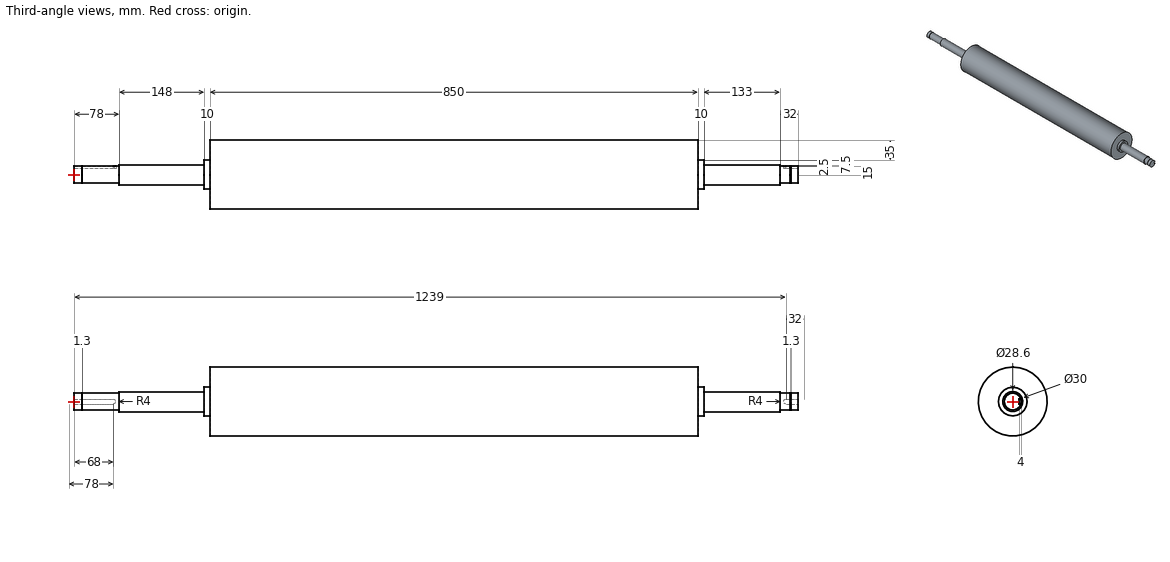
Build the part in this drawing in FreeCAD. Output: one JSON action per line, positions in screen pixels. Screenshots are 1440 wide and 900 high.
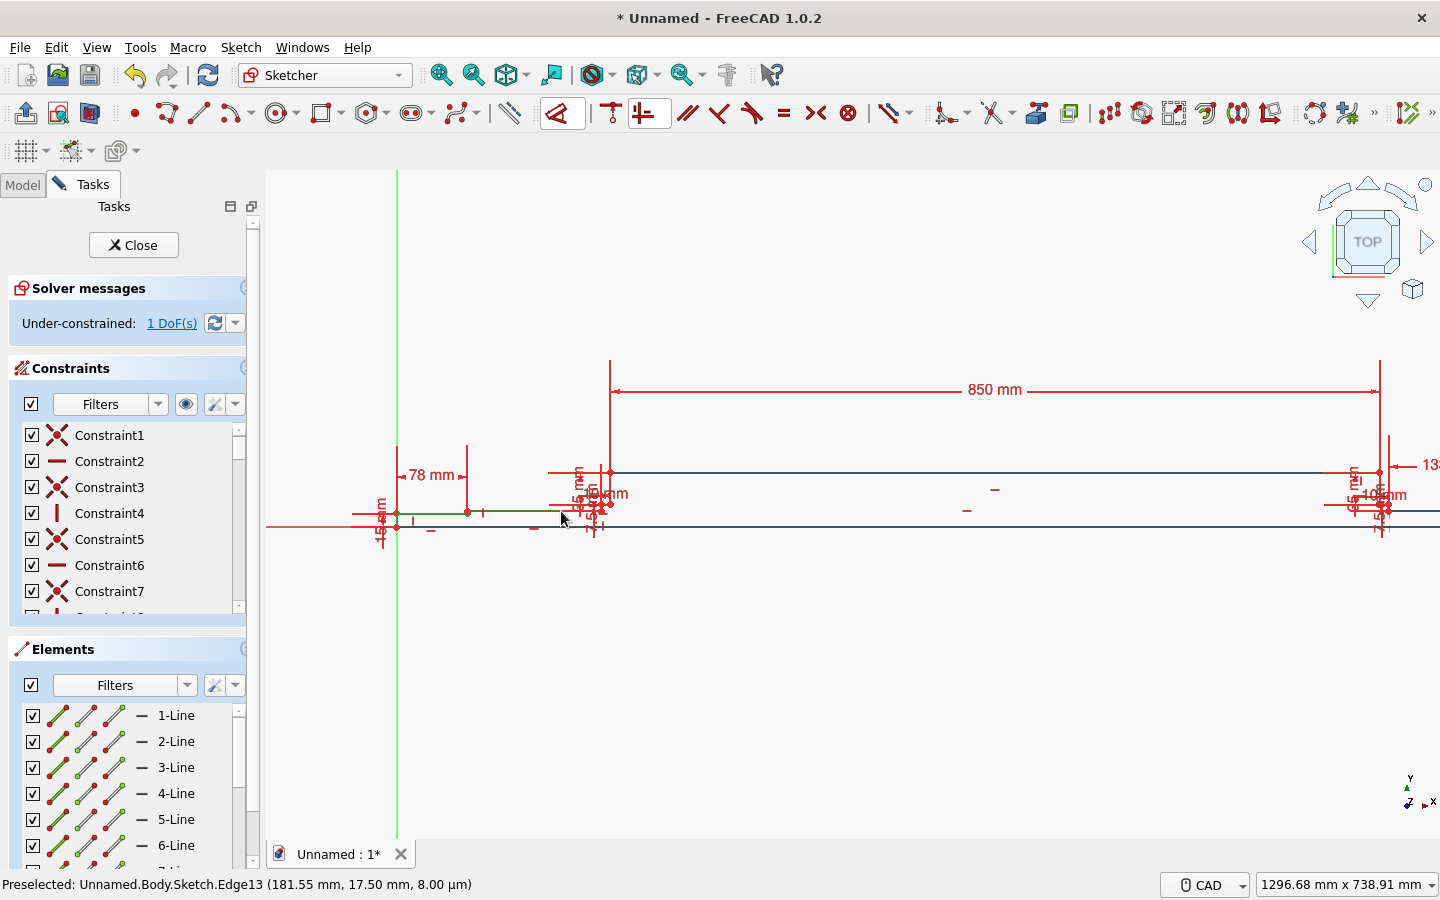
{"action": "key", "text": "l"}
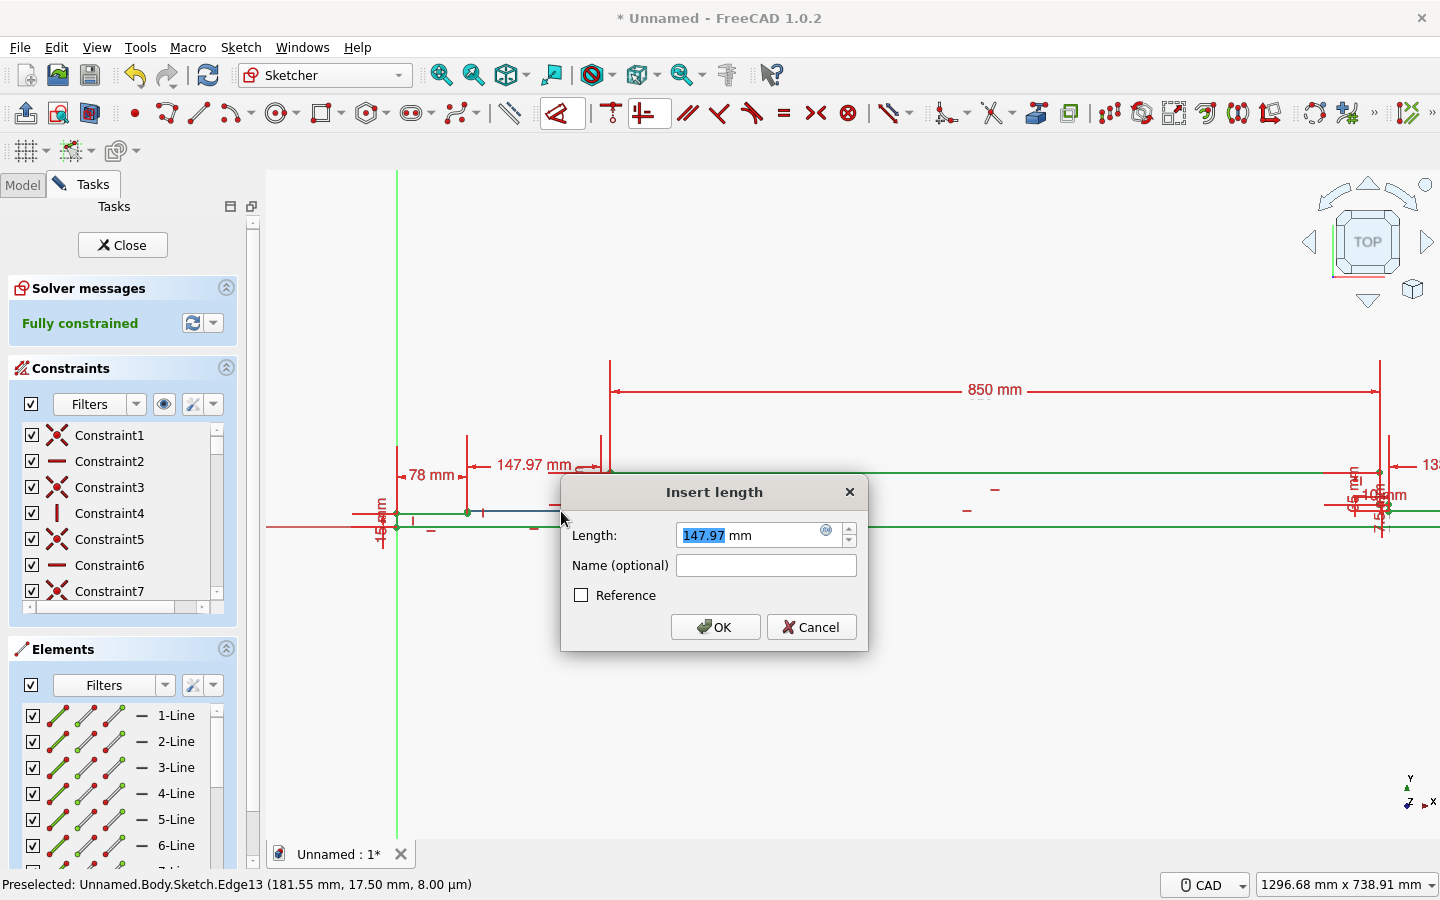
{"action": "type", "text": "148"}
{"action": "key", "text": "Return"}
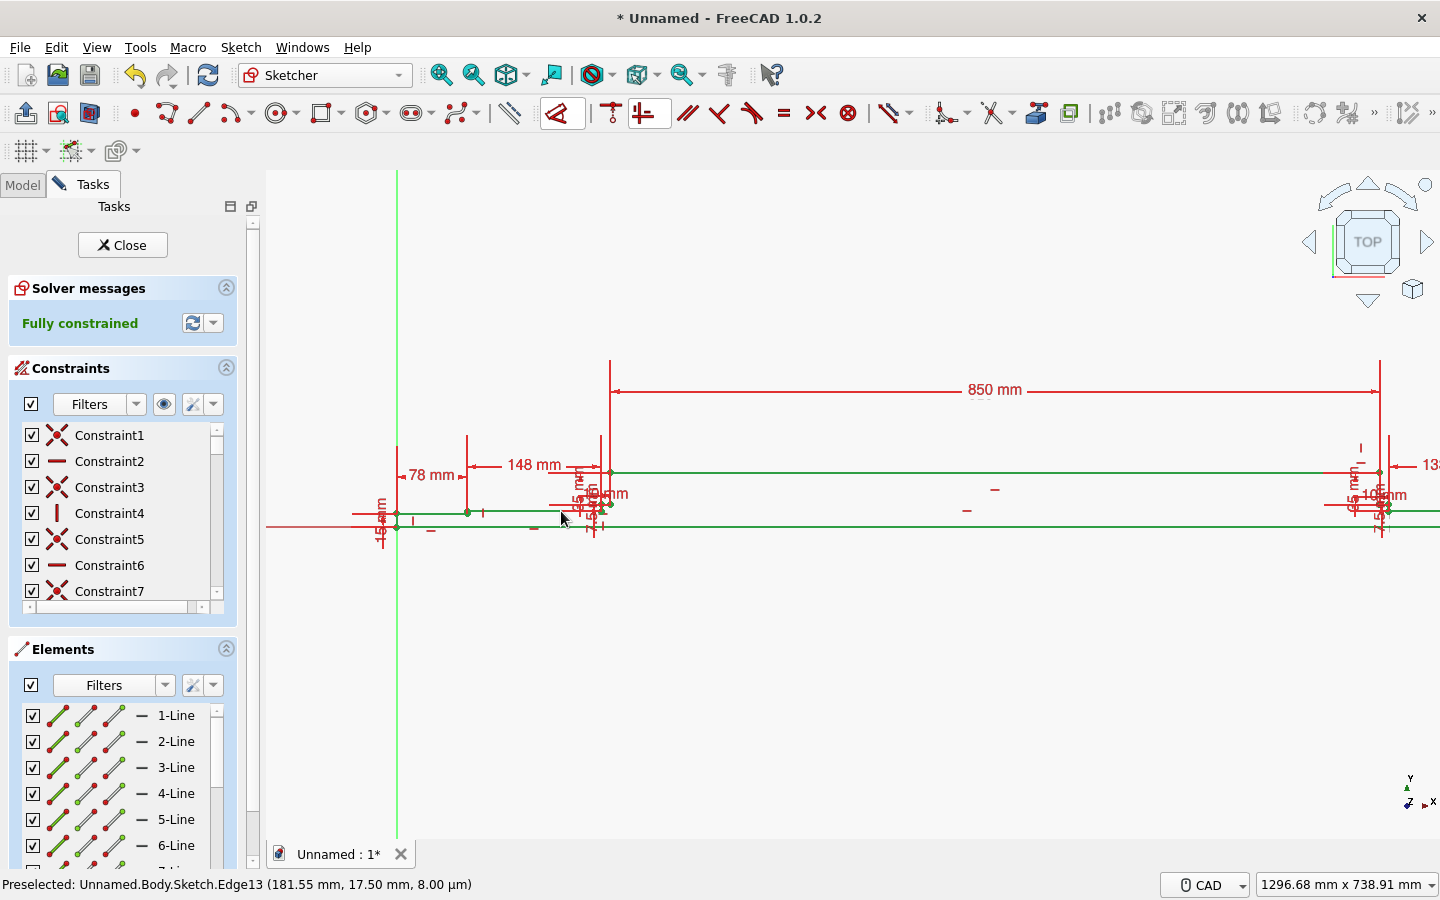
{"action": "left_click", "coordinate": [123, 245]}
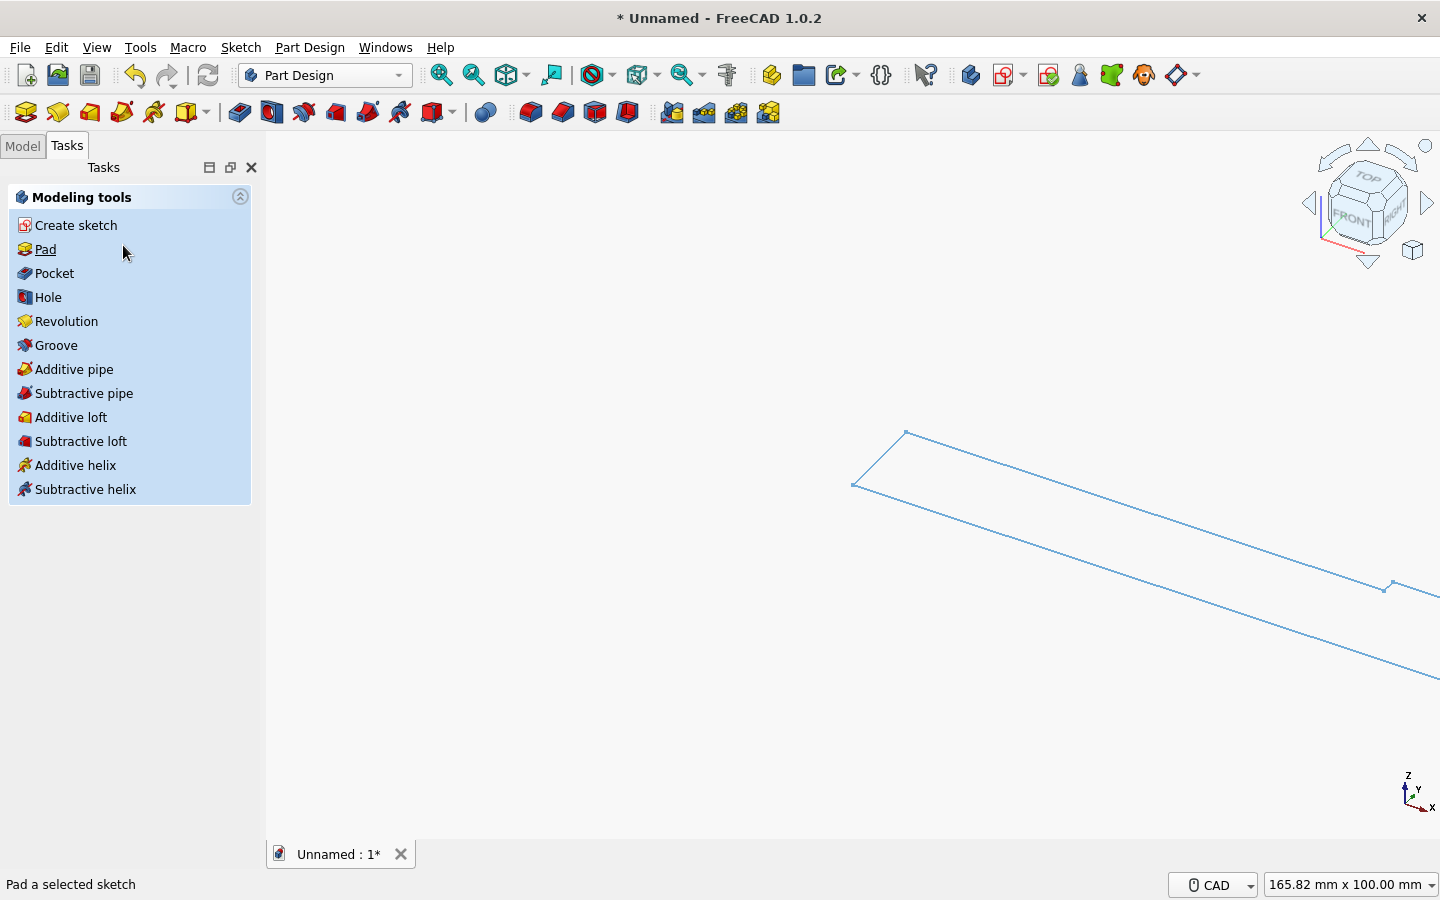
{"action": "left_click", "coordinate": [58, 112]}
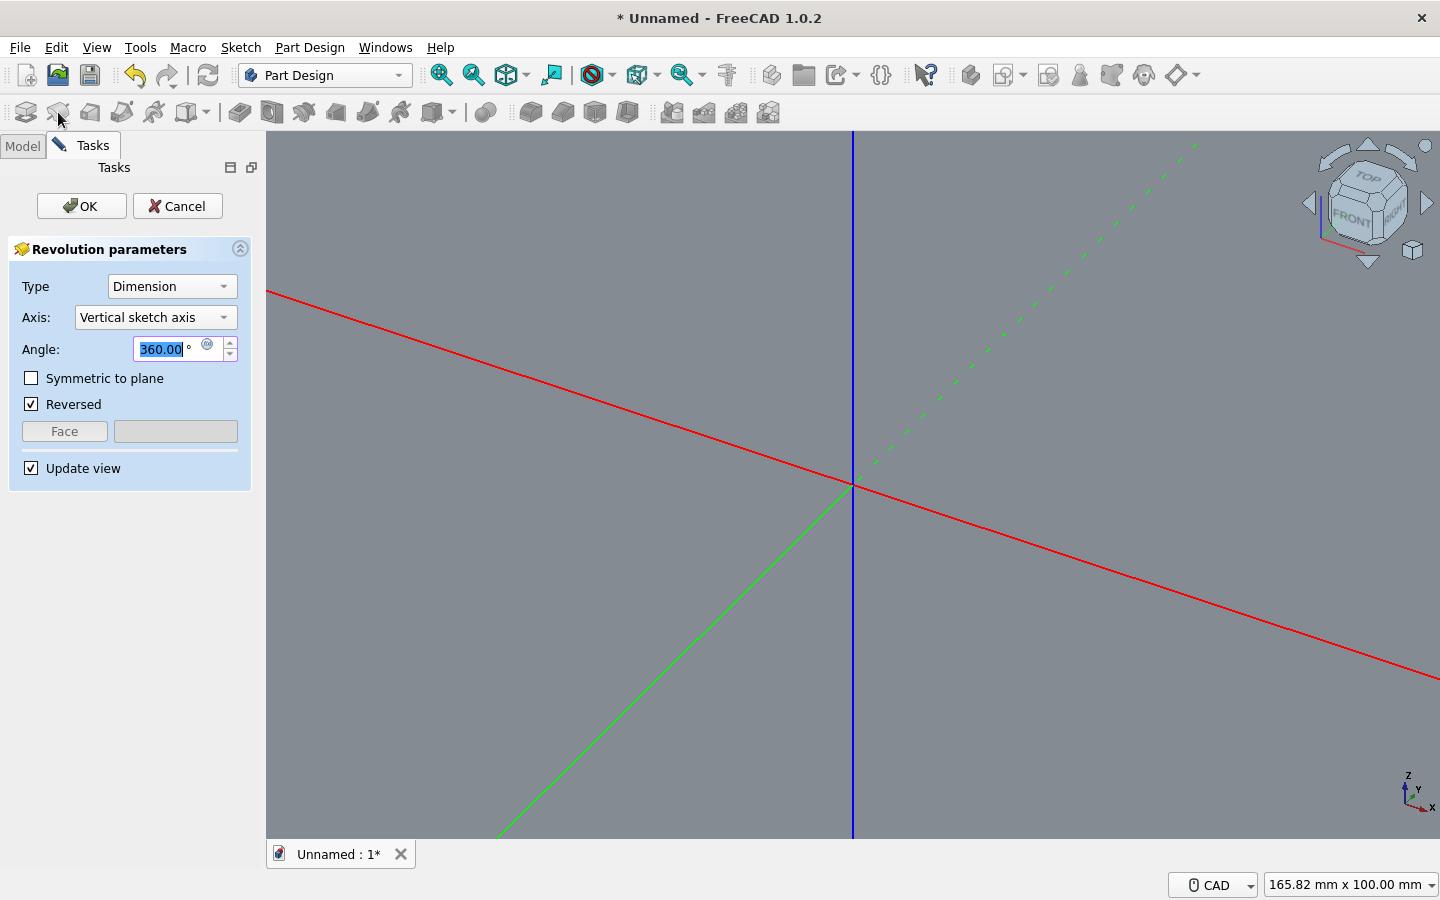
{"action": "left_click", "coordinate": [156, 318]}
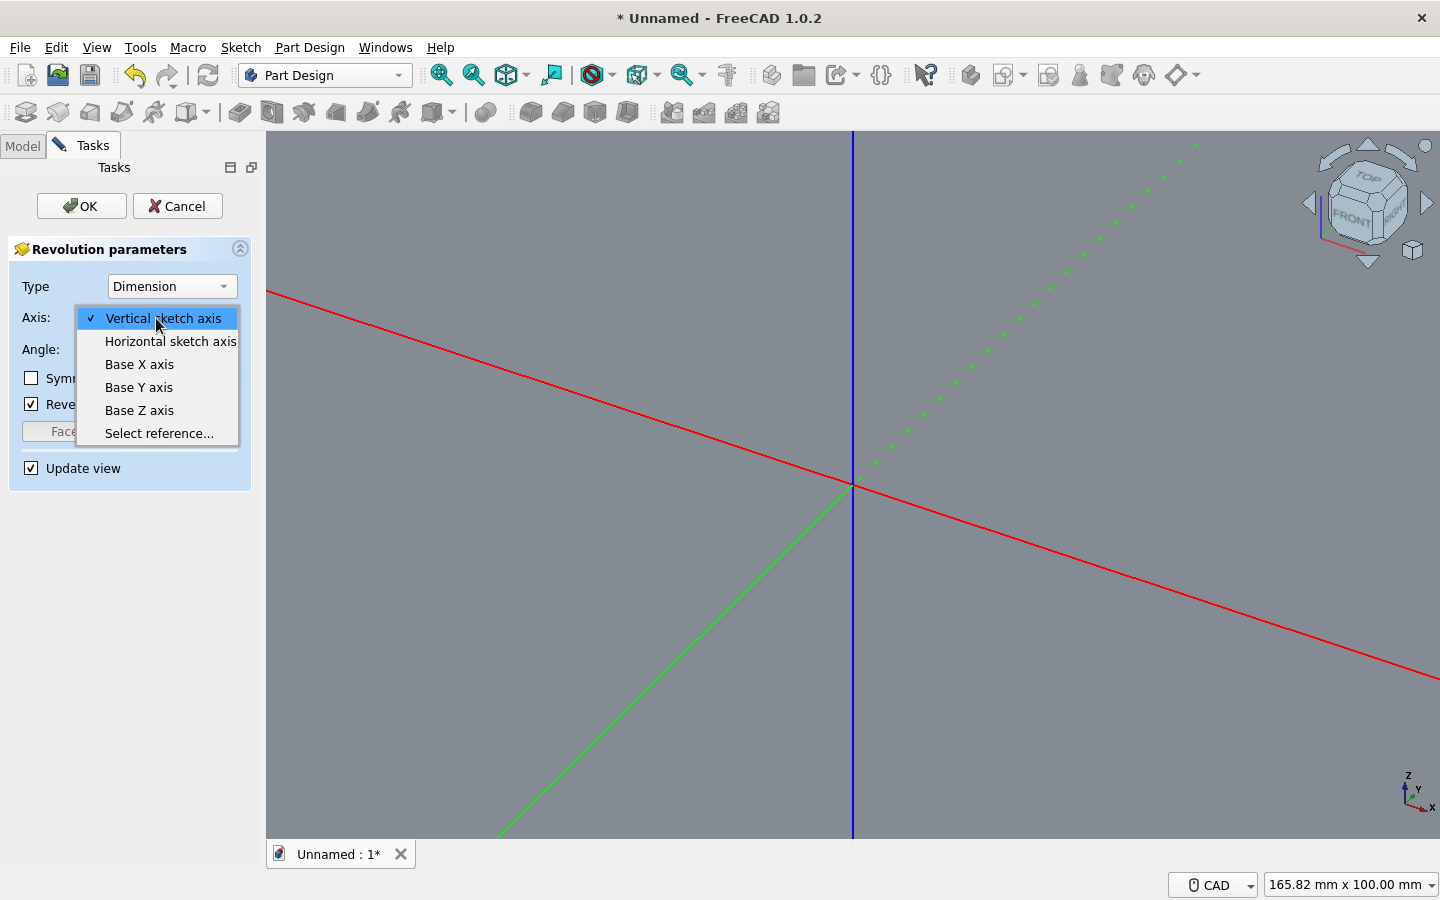
{"action": "left_click", "coordinate": [156, 342]}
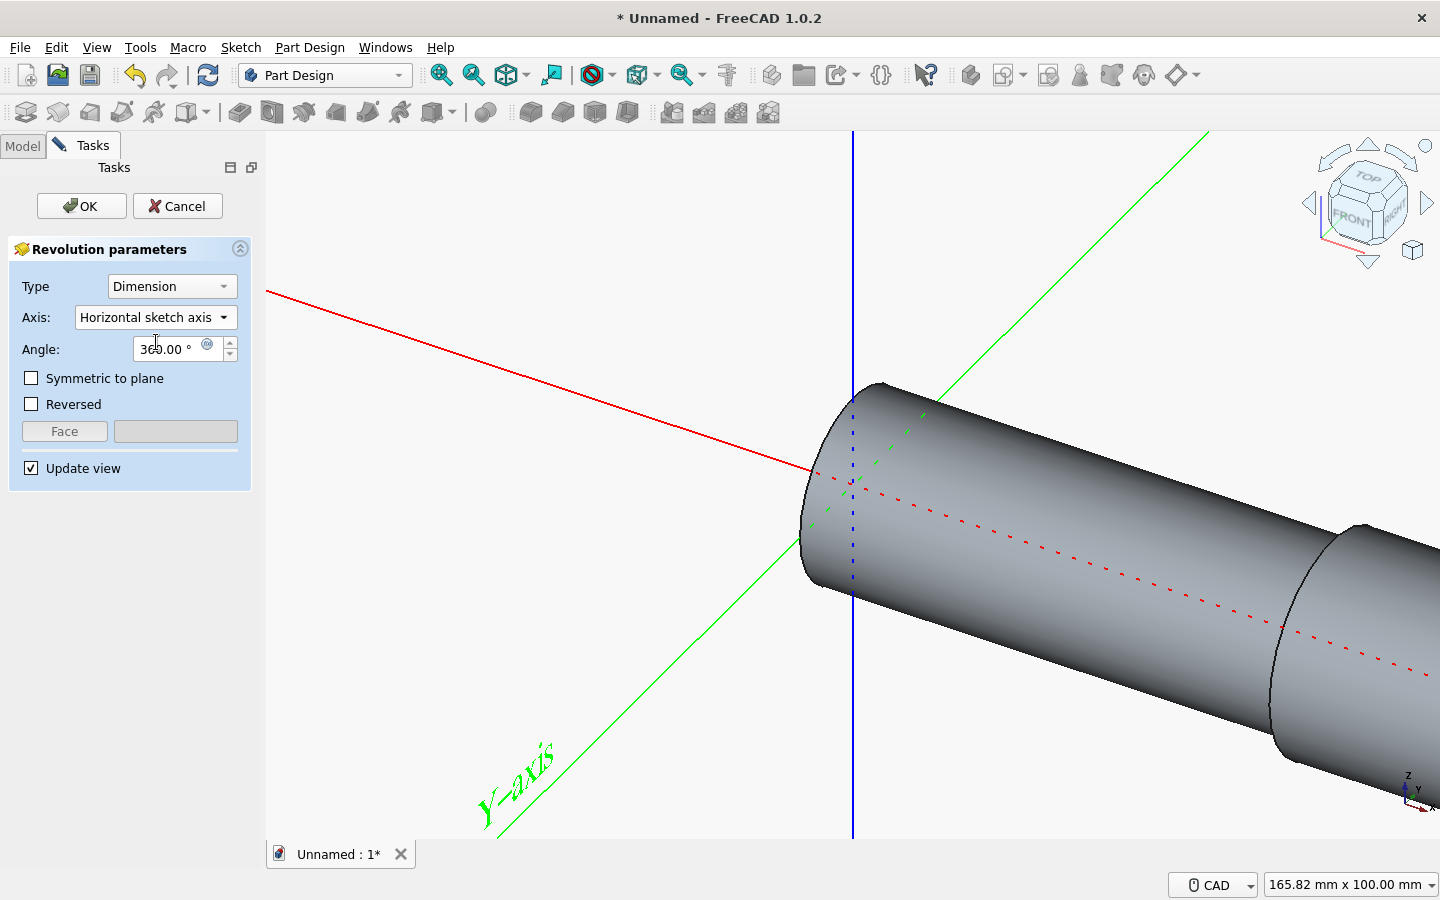
{"action": "left_click", "coordinate": [82, 206]}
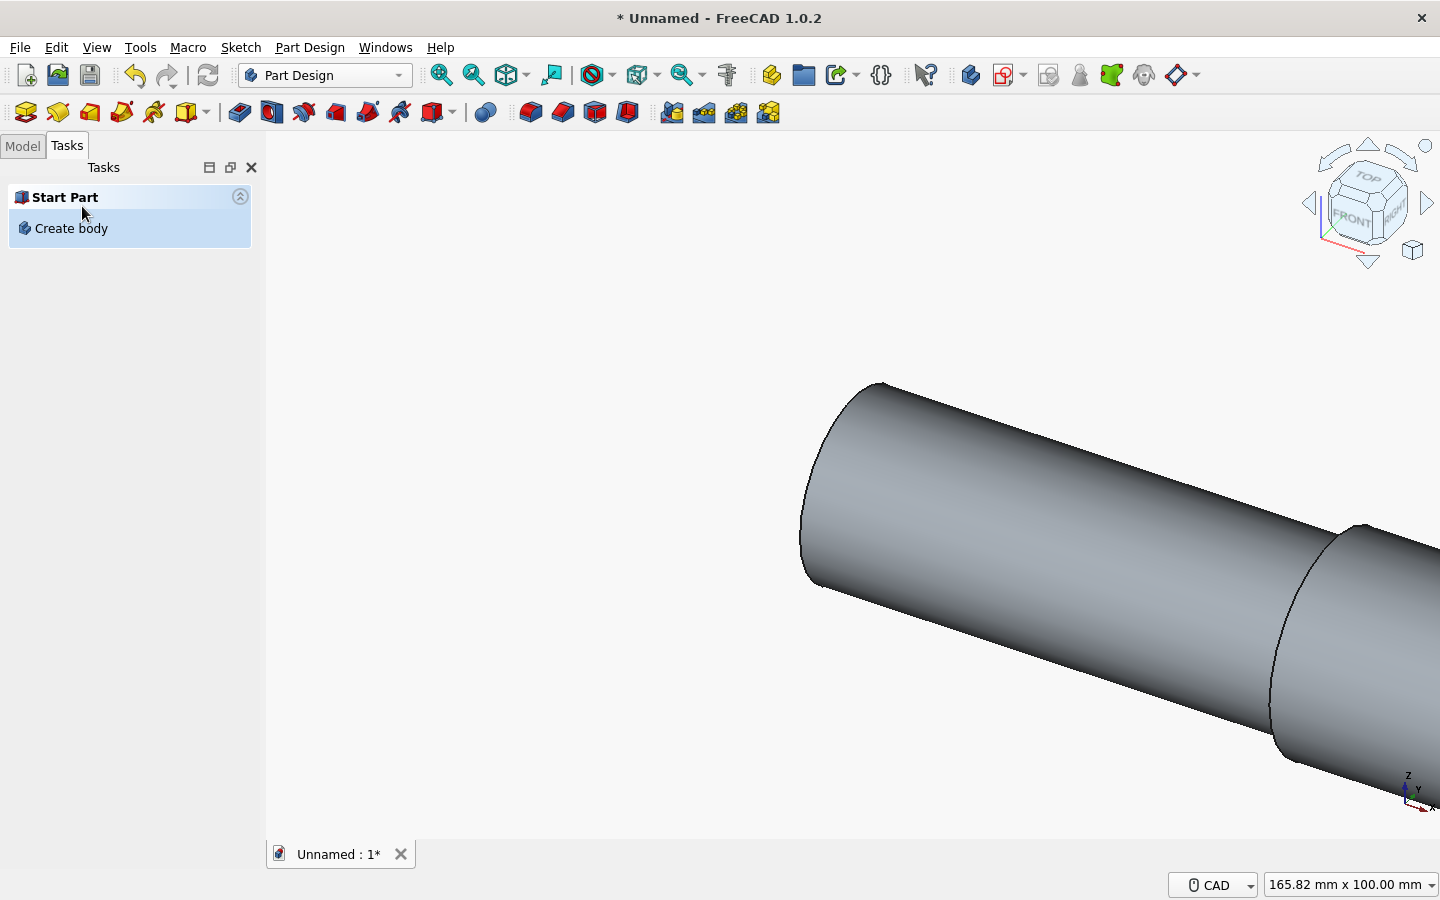
{"action": "key", "text": "v f"}